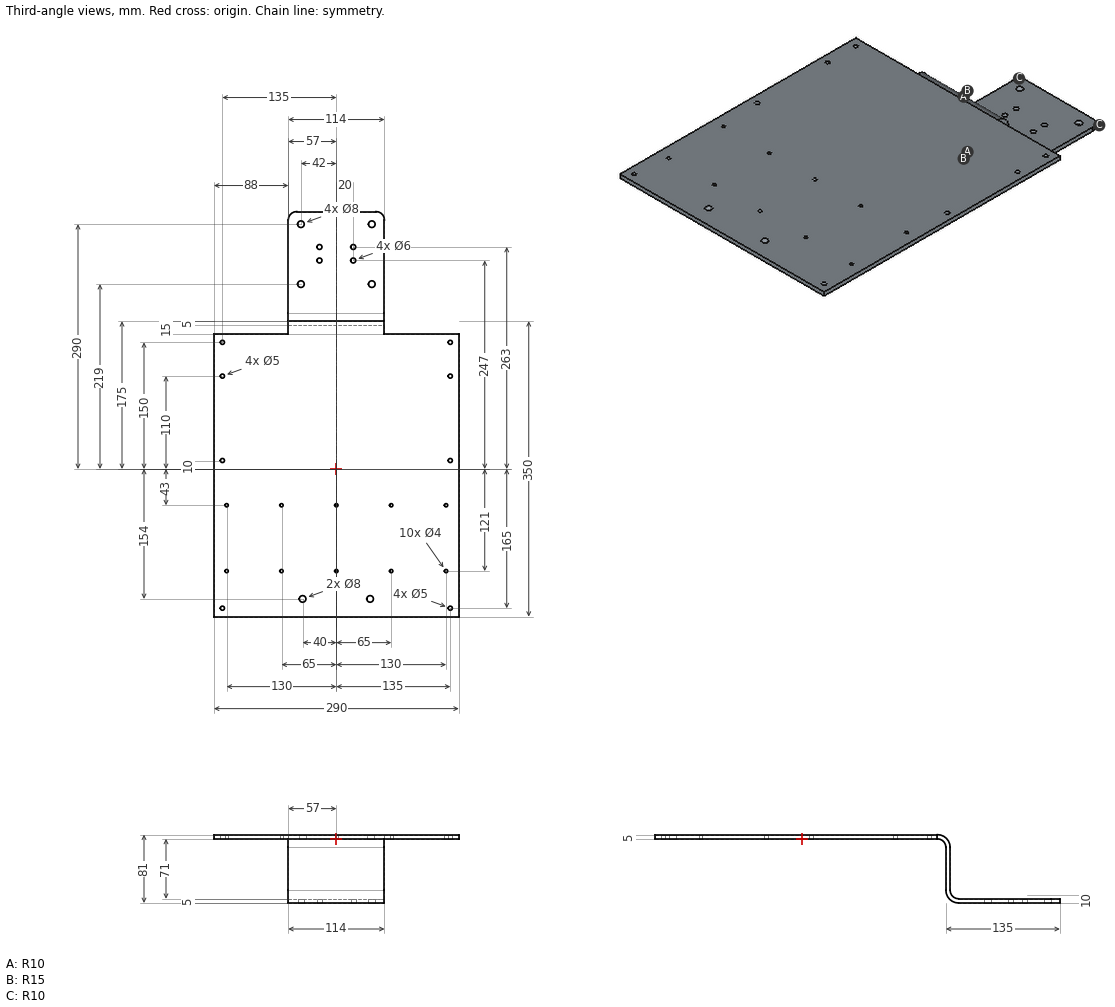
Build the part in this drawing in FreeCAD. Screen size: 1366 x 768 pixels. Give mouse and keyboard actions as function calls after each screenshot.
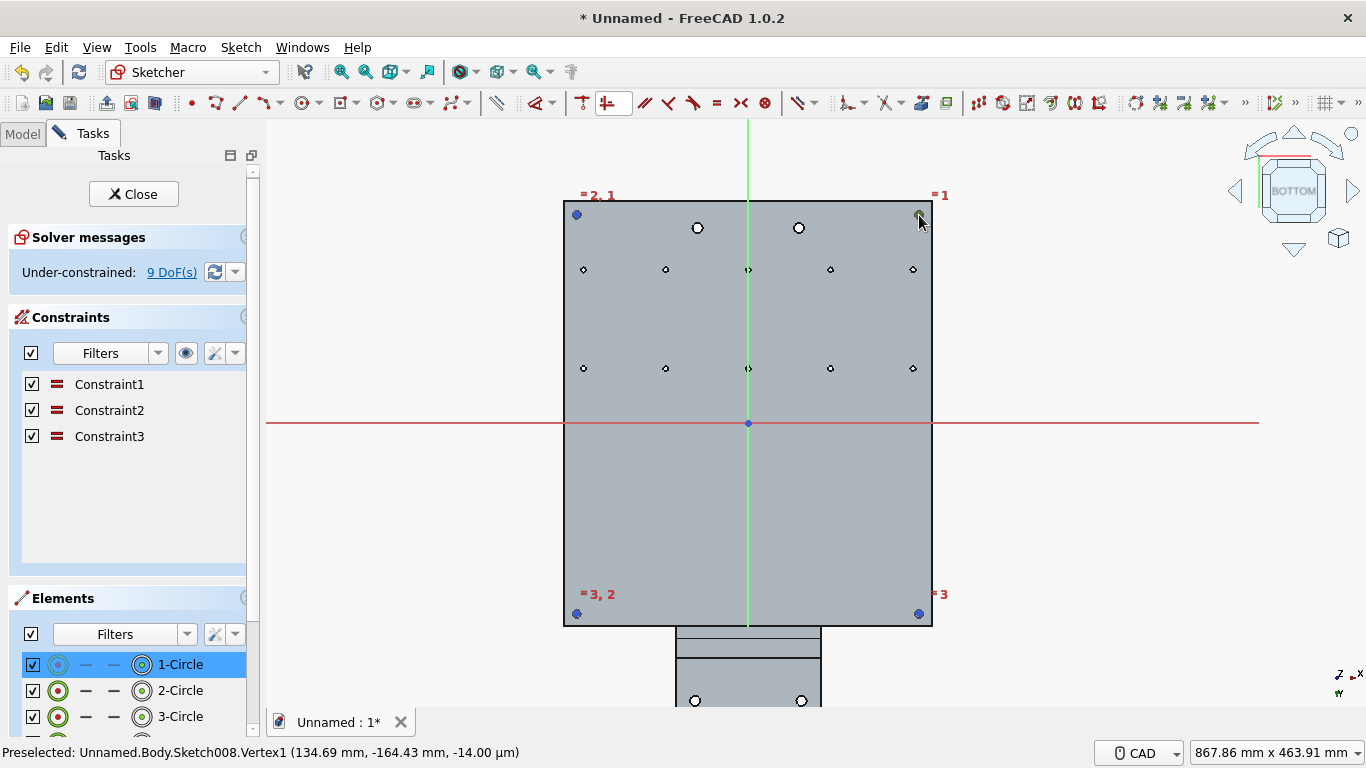
click(577, 215)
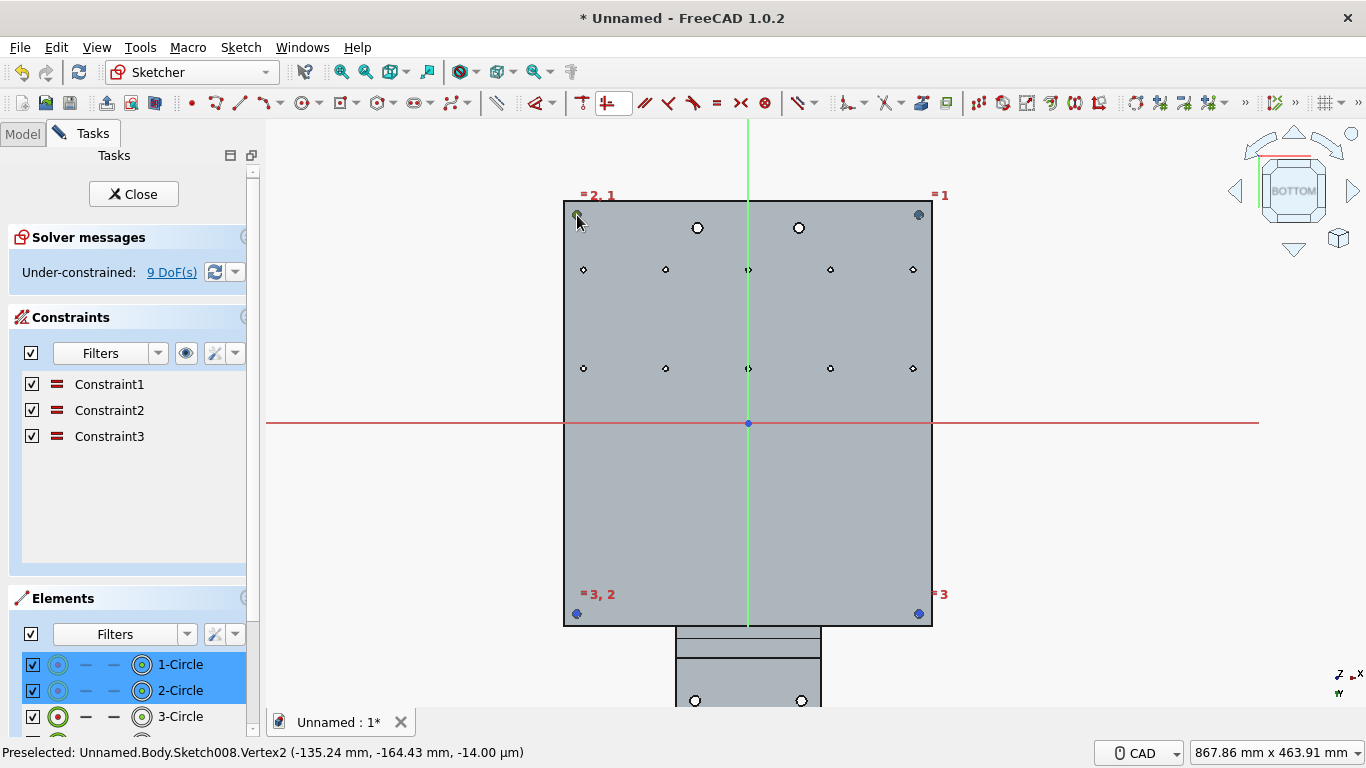
click(748, 641)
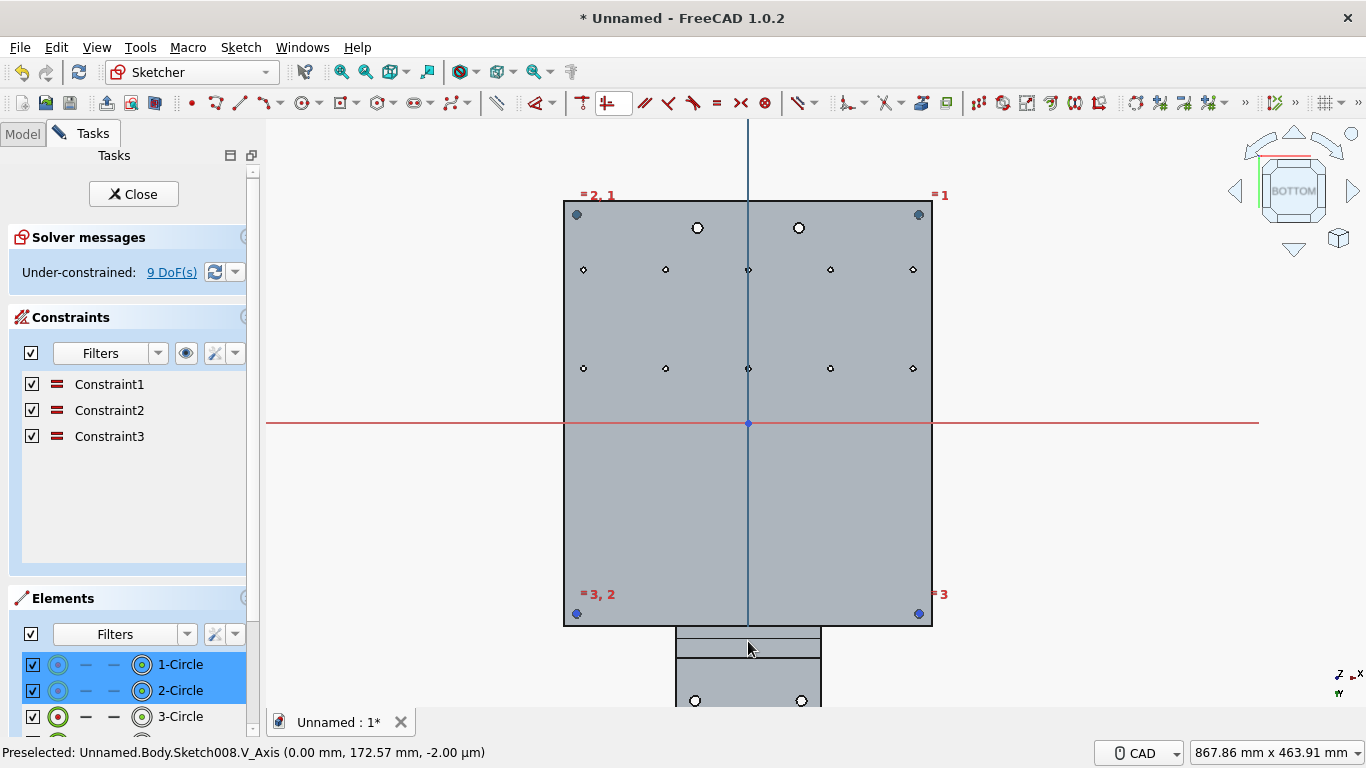
click(742, 104)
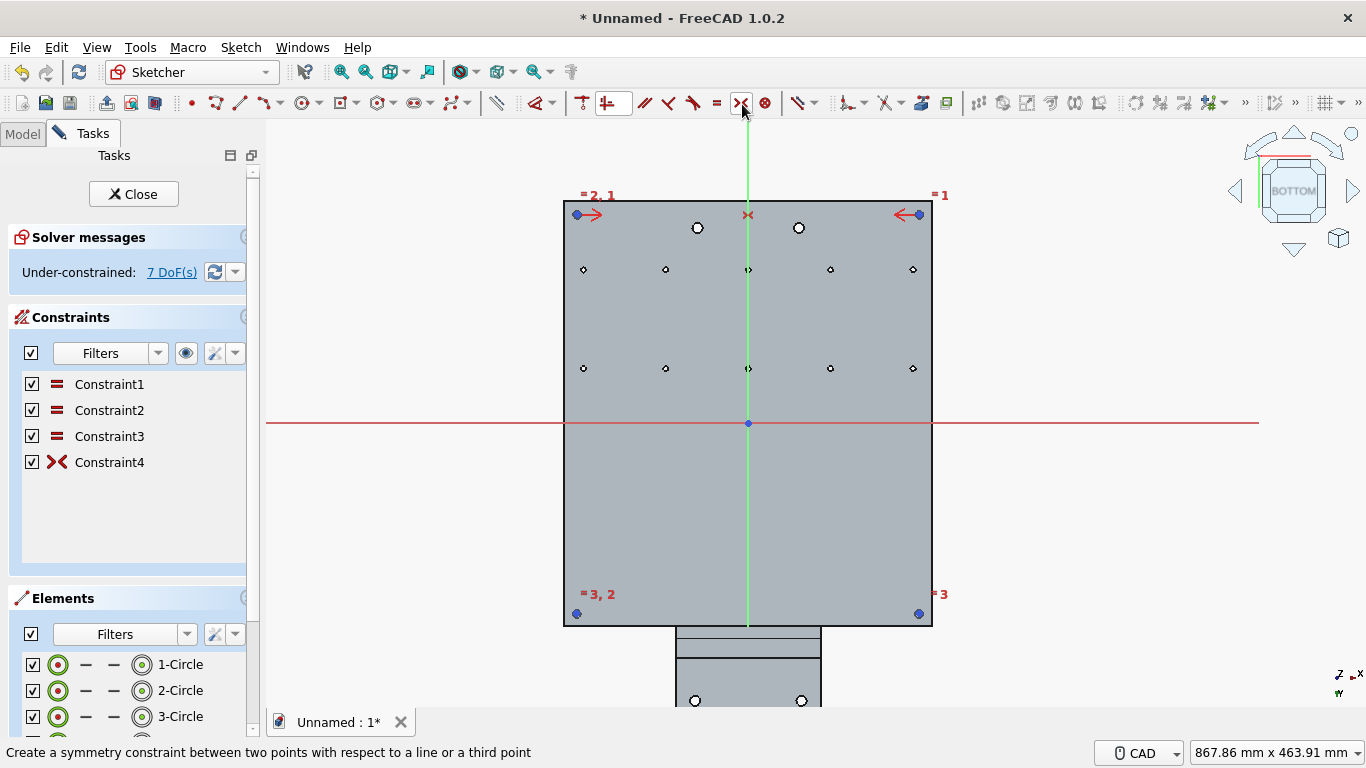
click(577, 614)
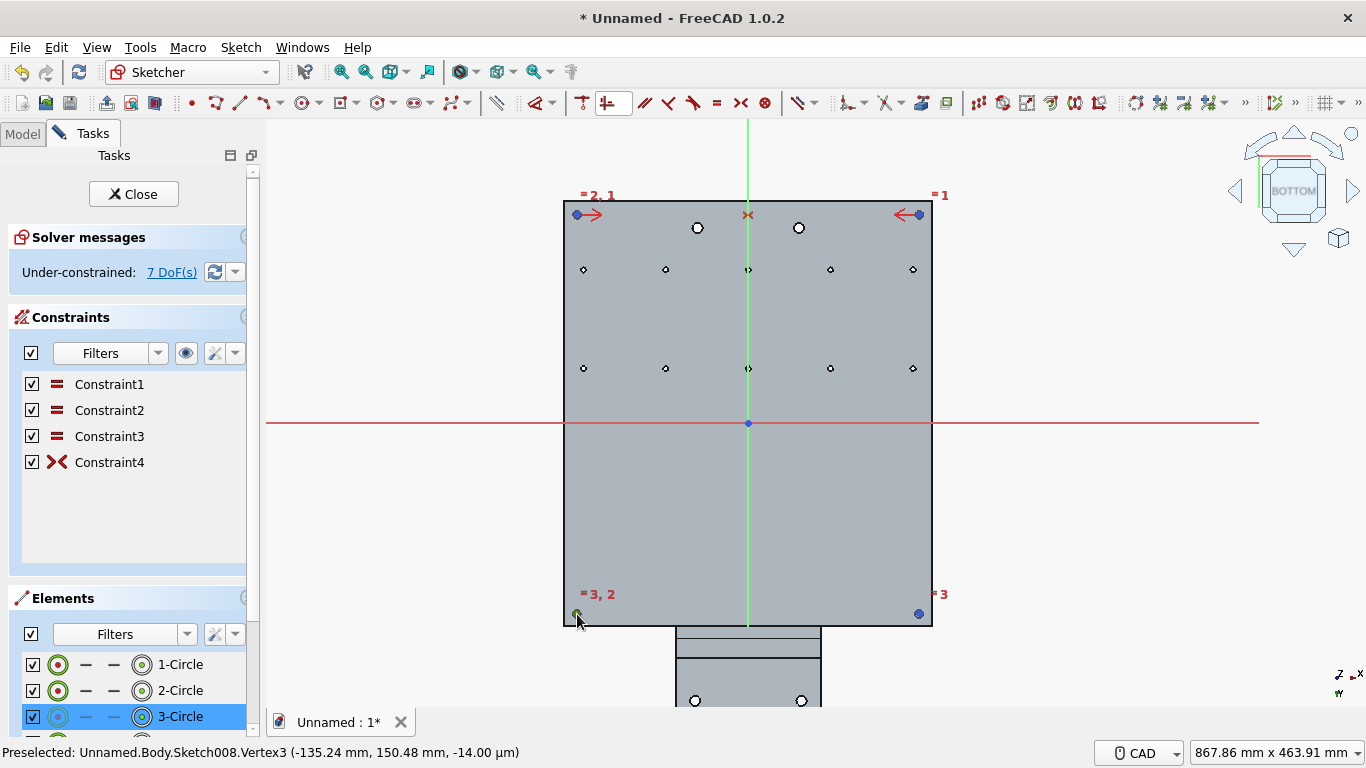
click(919, 614)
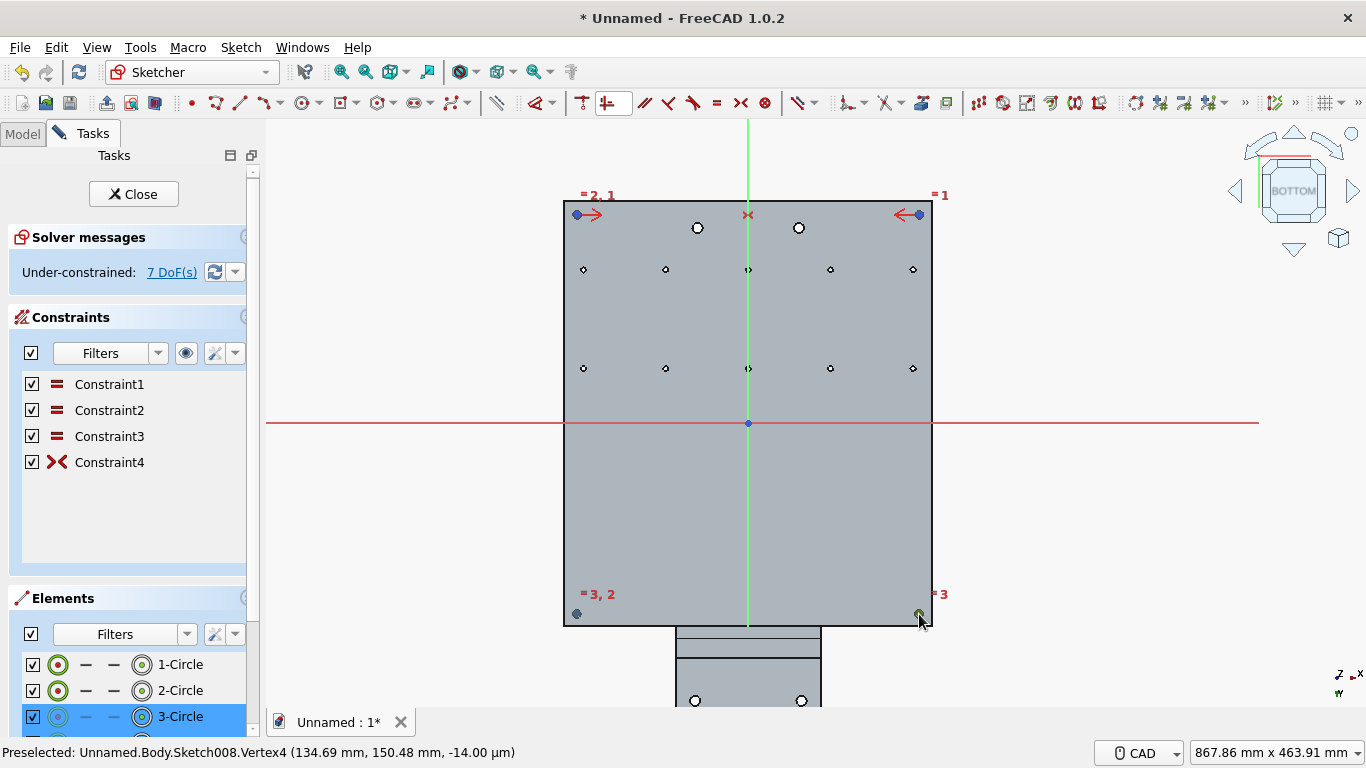
click(748, 641)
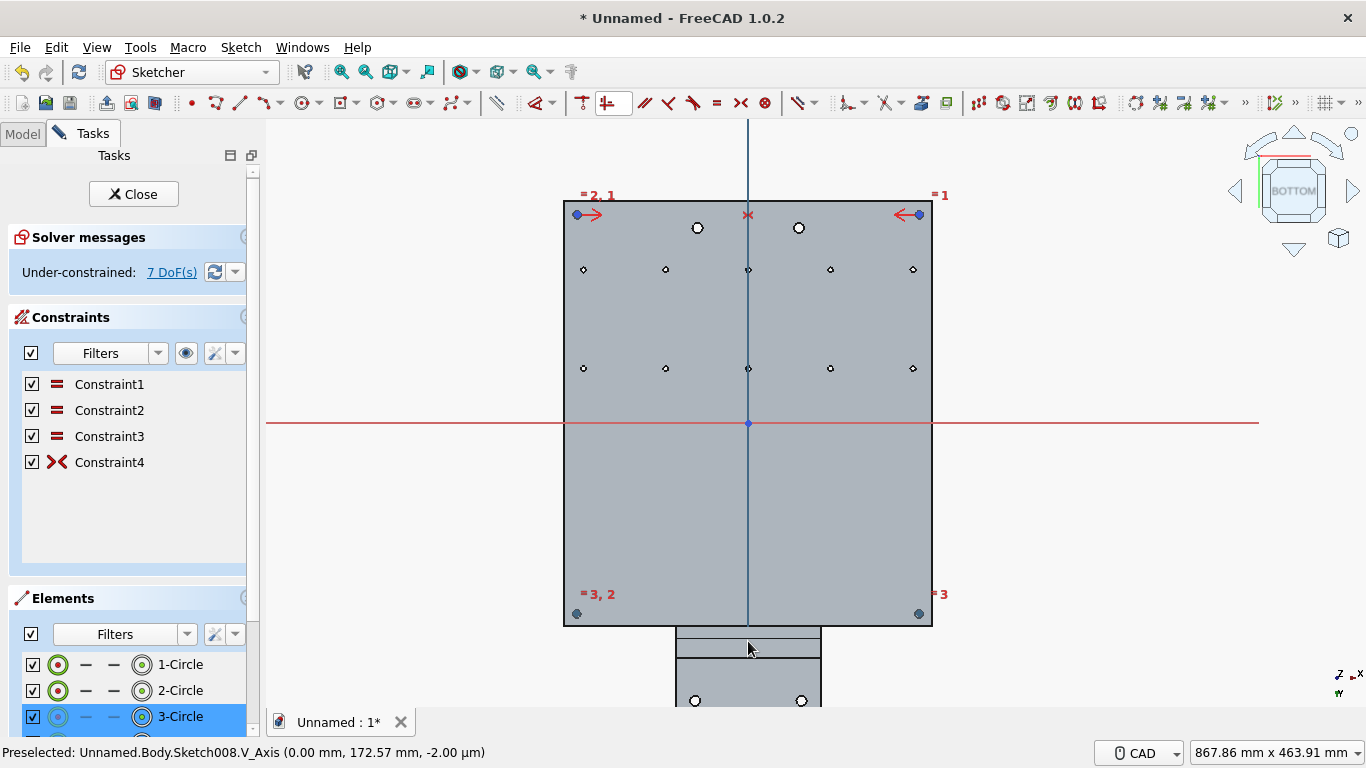
click(742, 104)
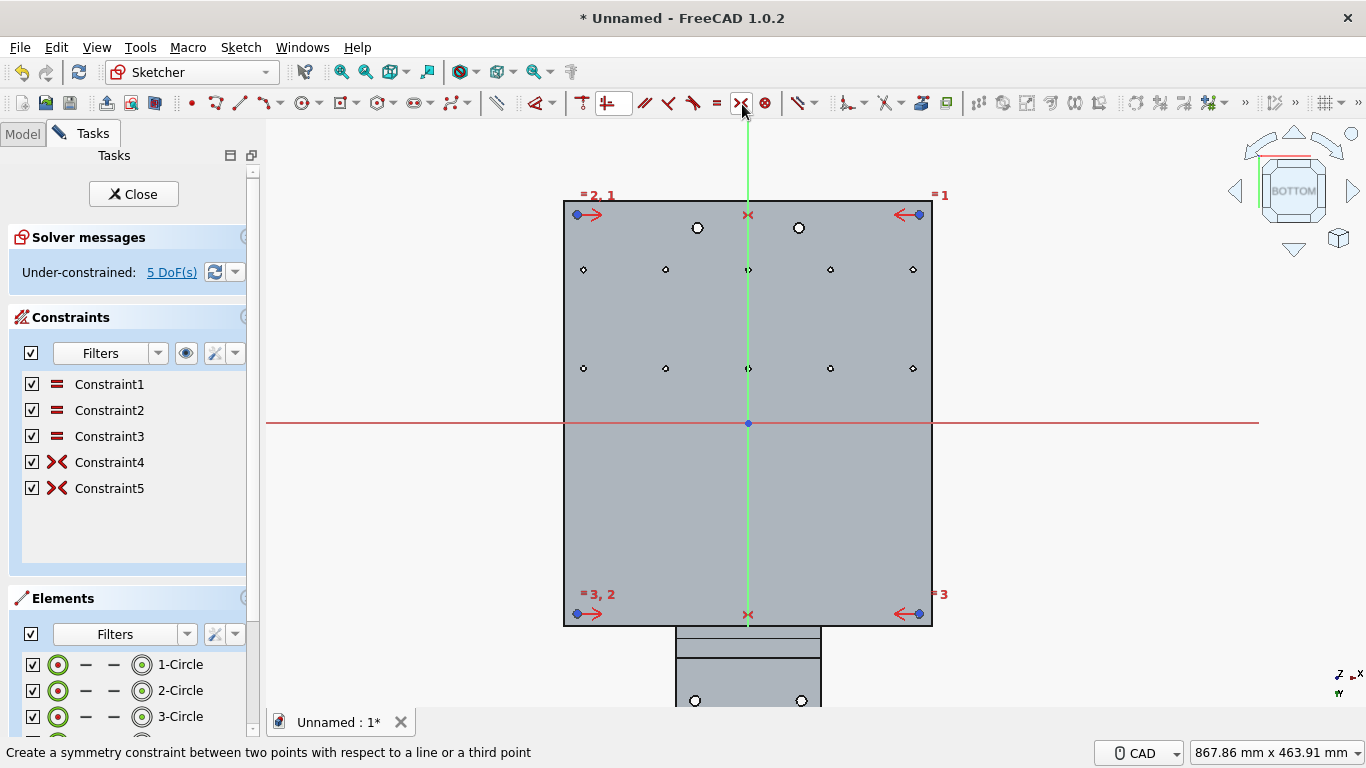
click(536, 104)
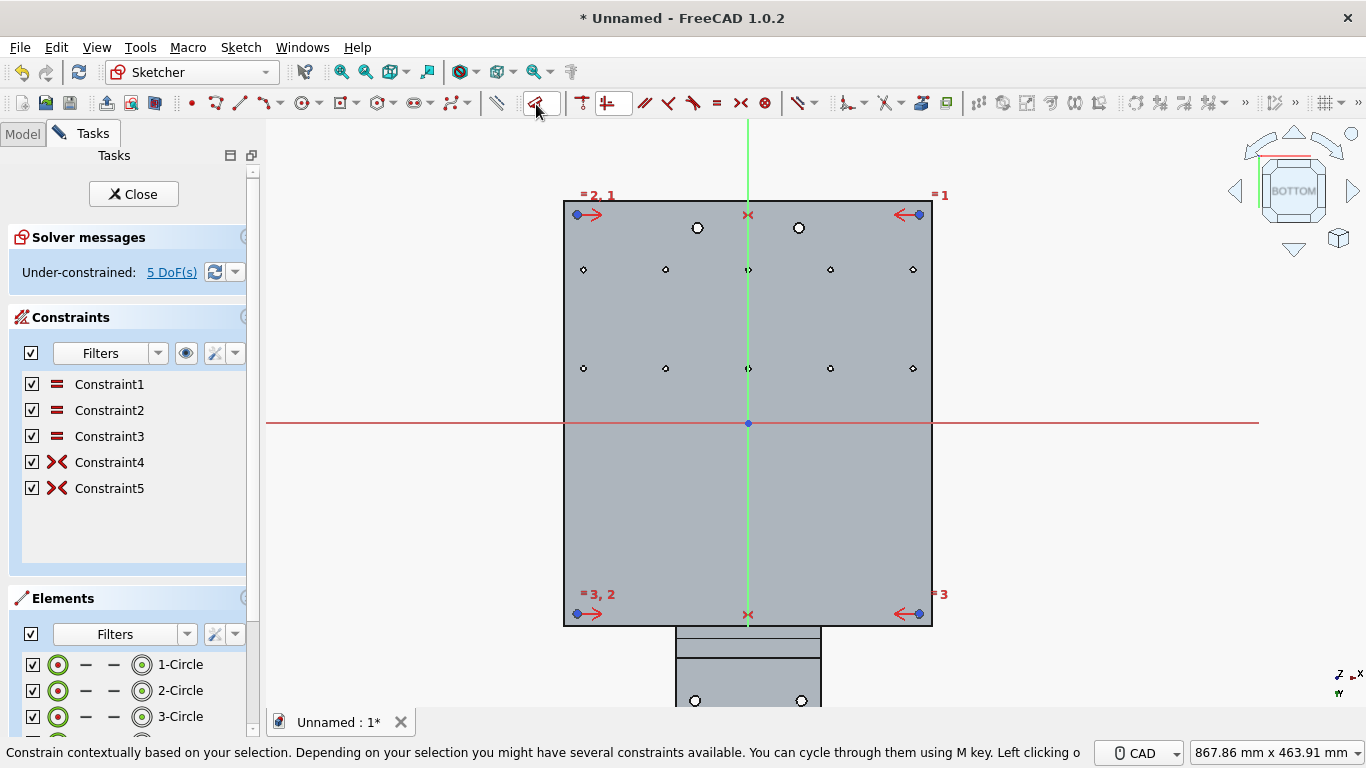
scroll(922, 212, up, 10)